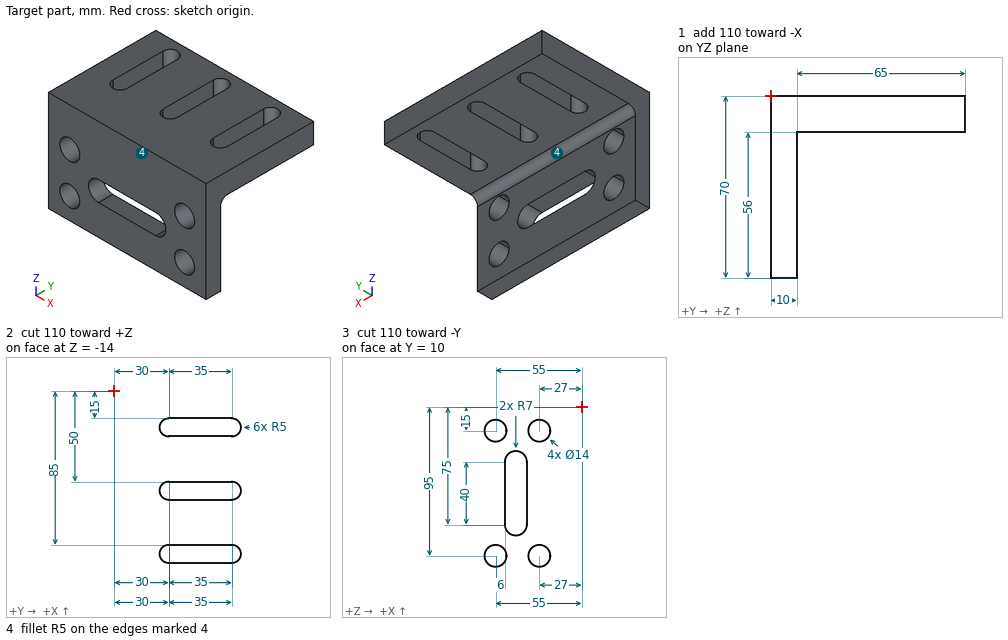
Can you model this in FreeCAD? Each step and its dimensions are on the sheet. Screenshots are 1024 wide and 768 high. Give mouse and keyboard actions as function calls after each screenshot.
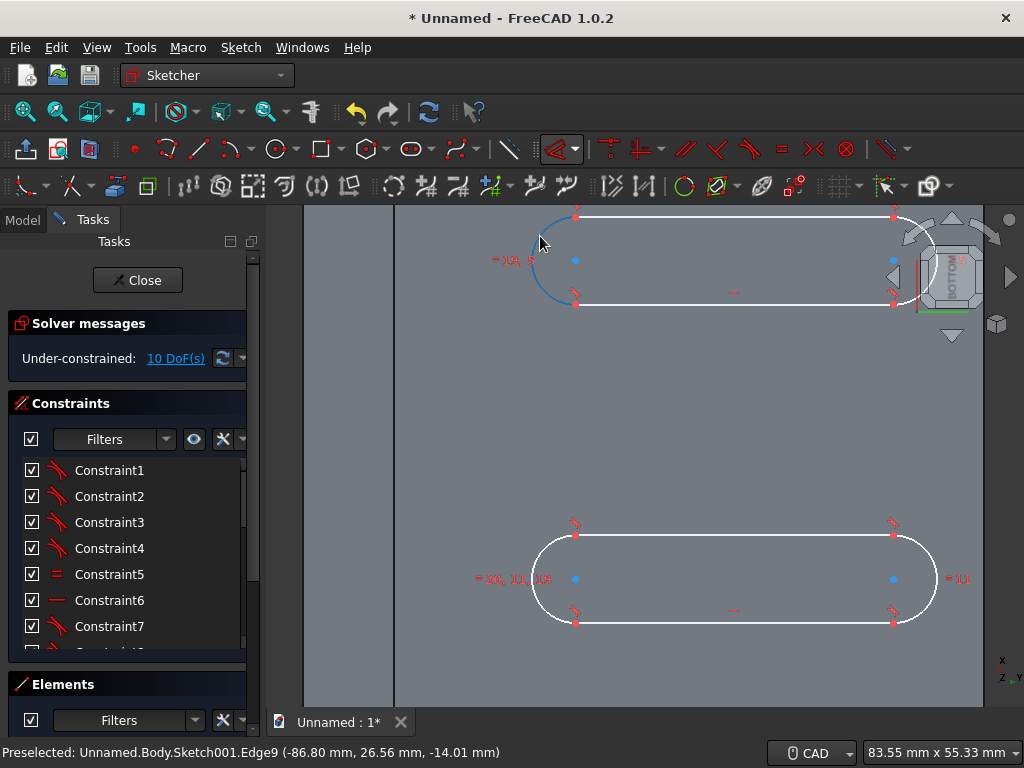
click(541, 235)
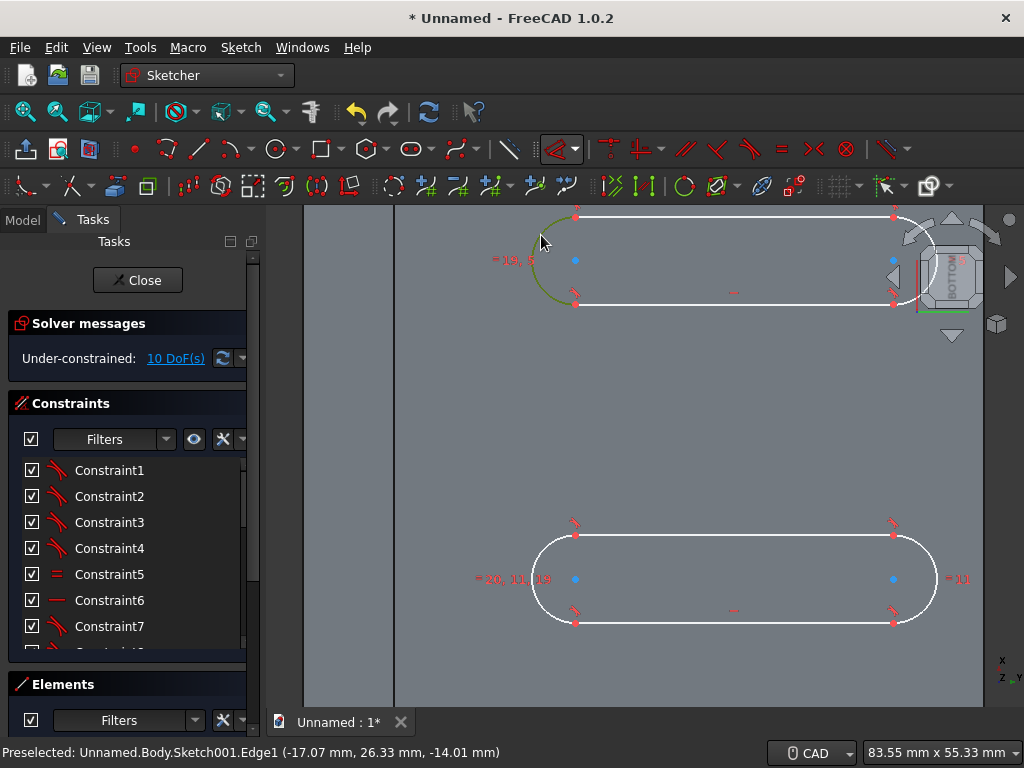
key(k)
key(r)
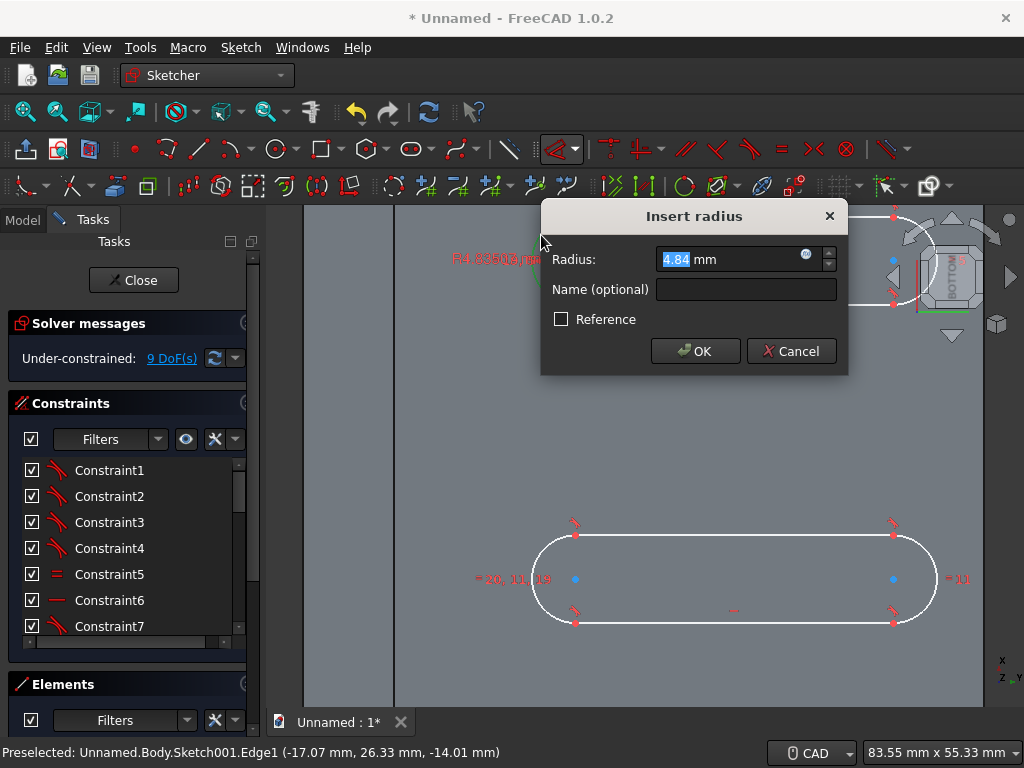
text(5)
key(Return)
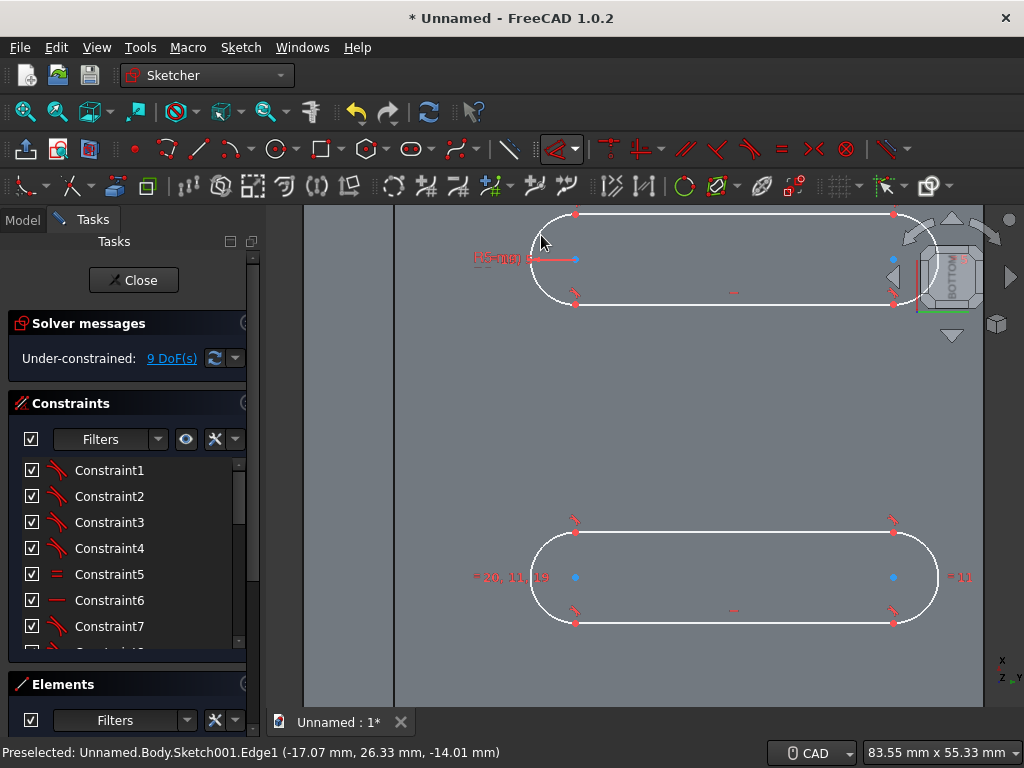
scroll(551, 425, down, 5)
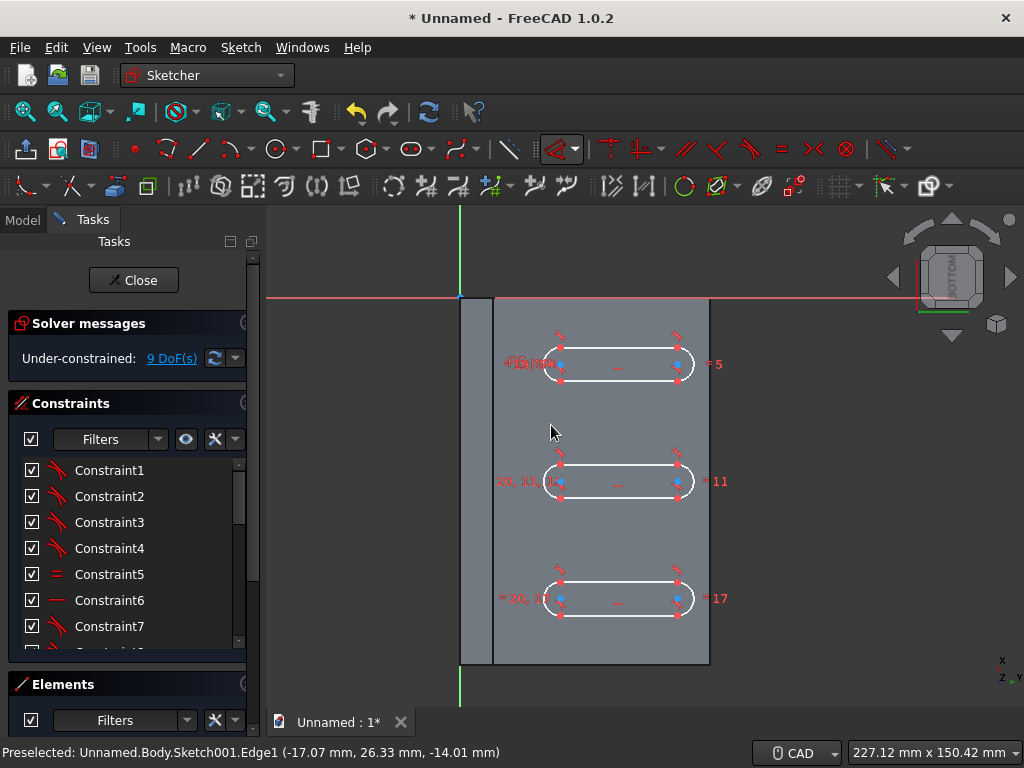
click(595, 348)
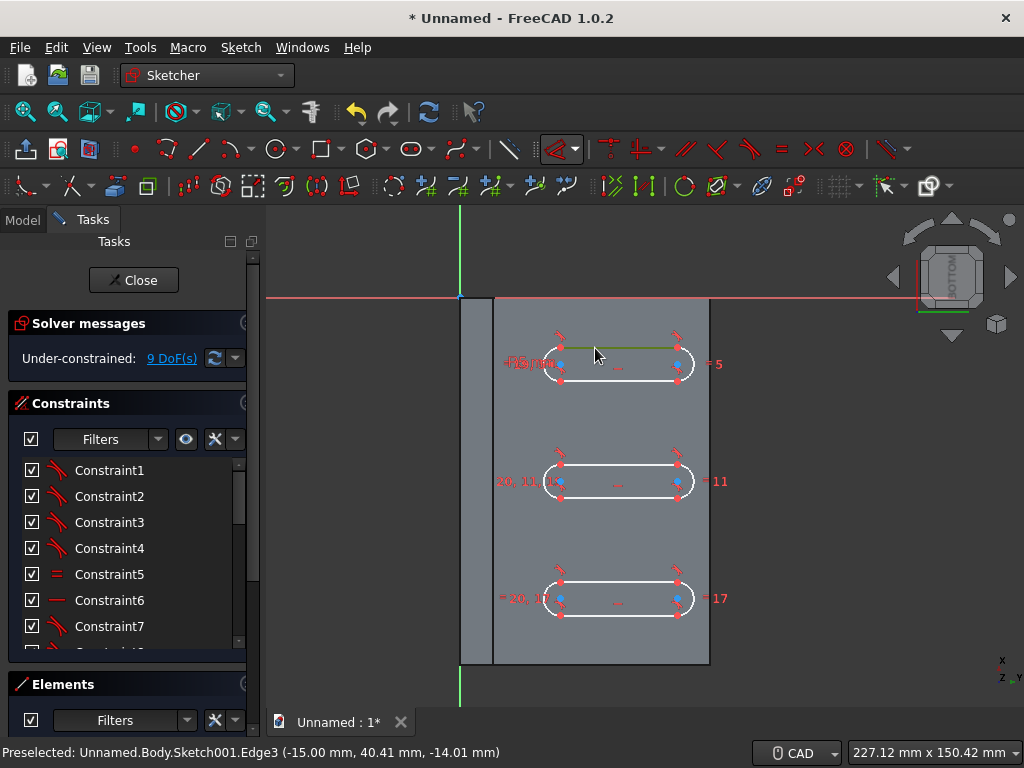
key(l)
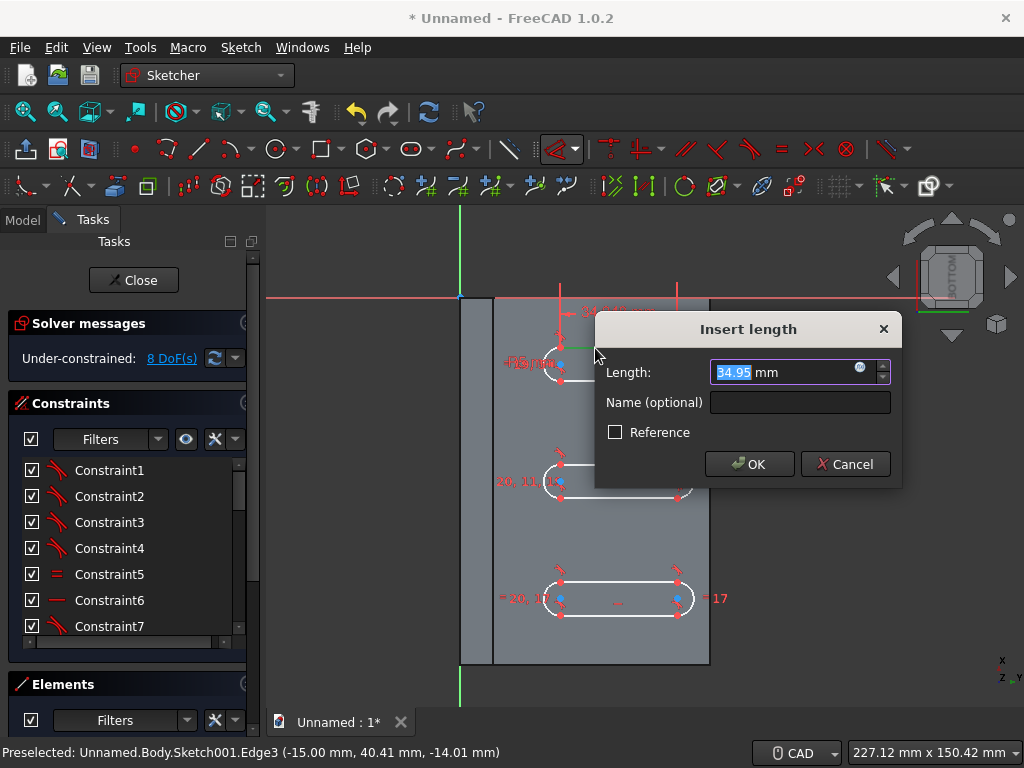
text(35)
key(Return)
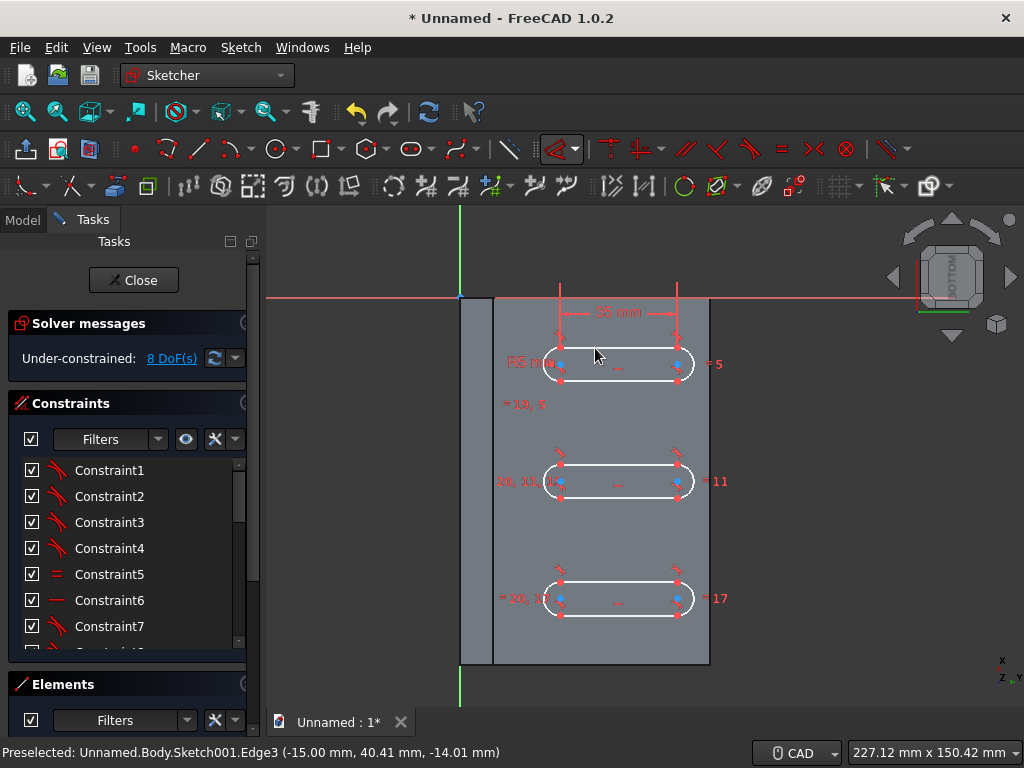
click(595, 465)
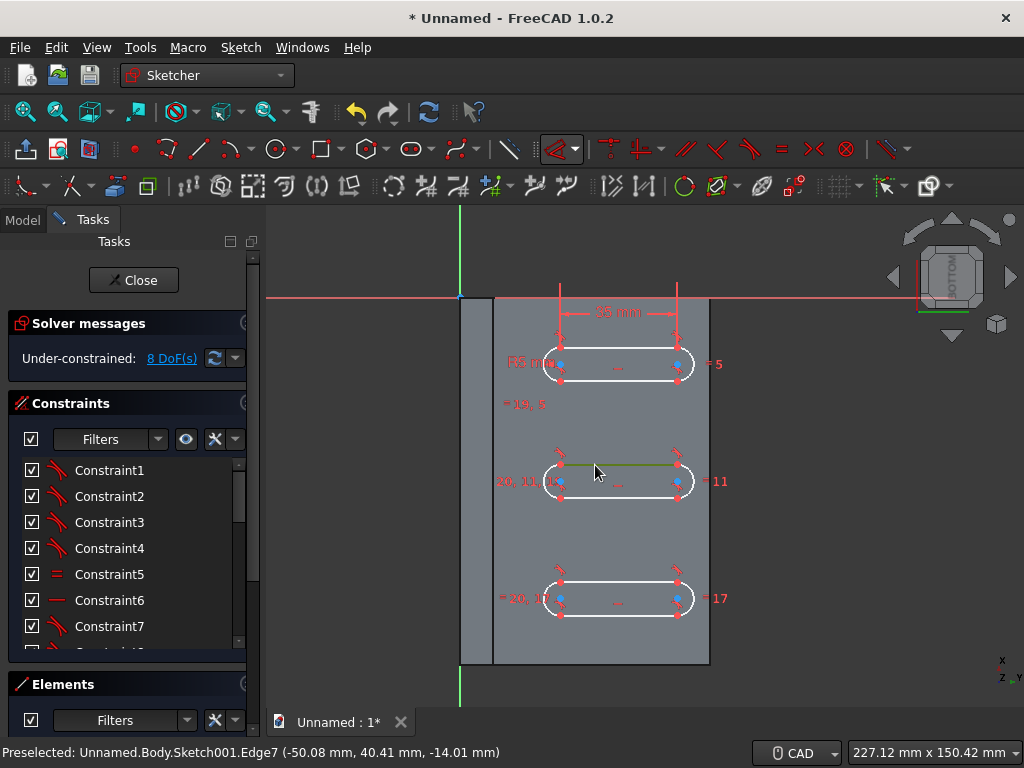
key(l)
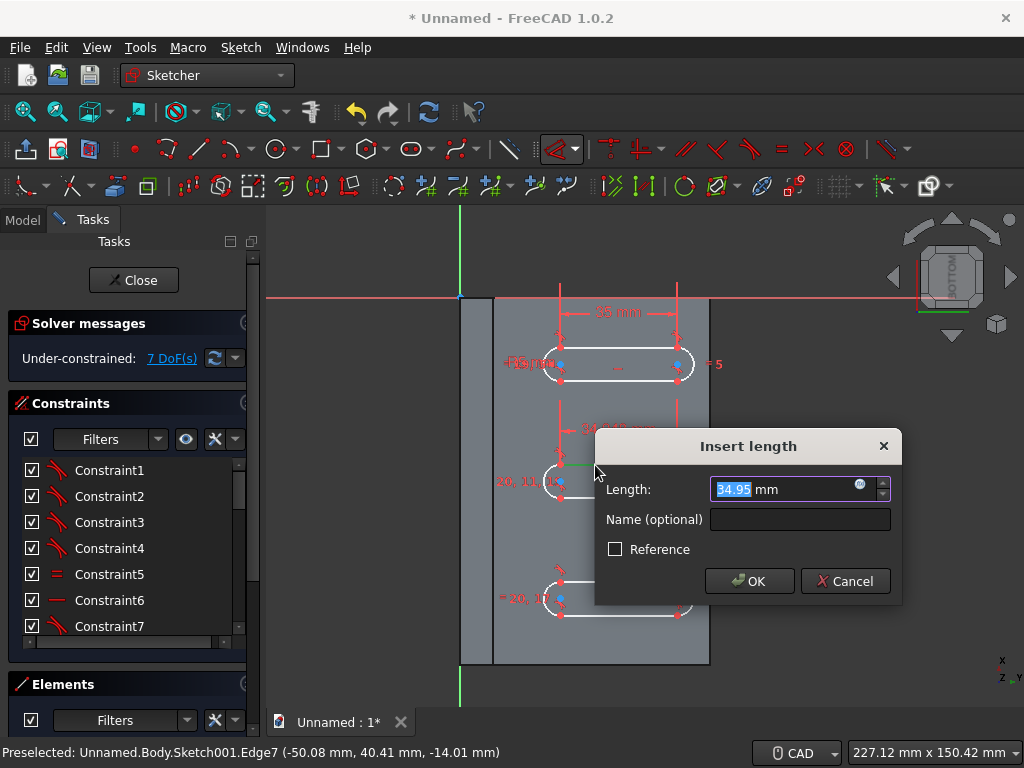
text(35)
key(Return)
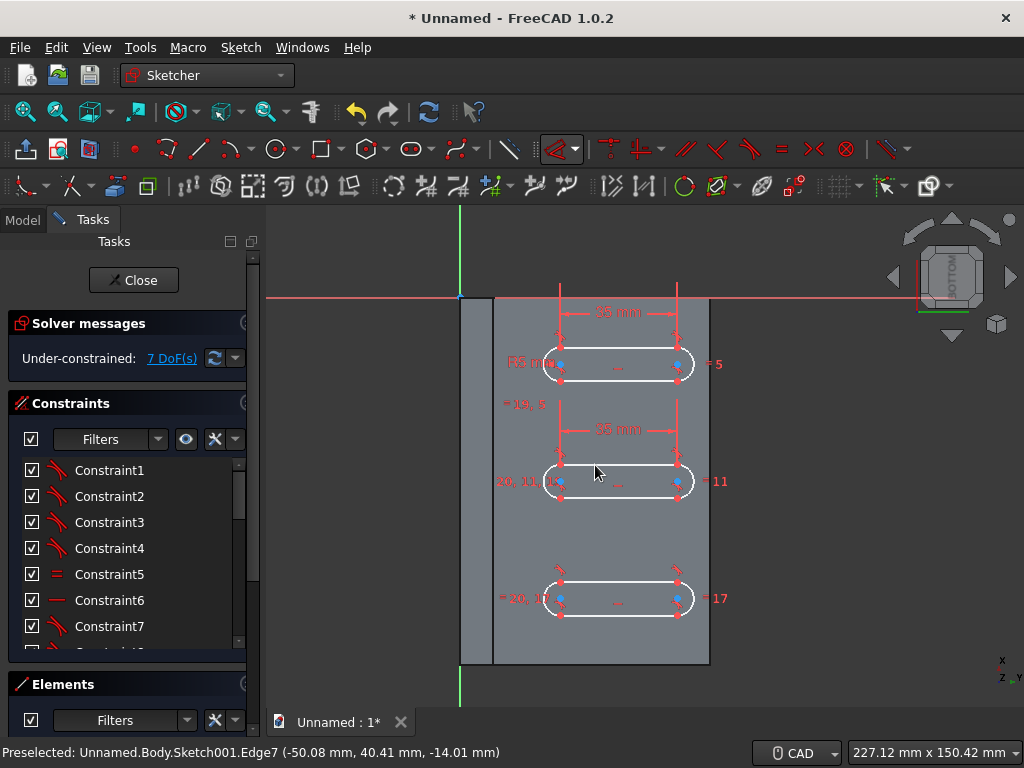
click(595, 582)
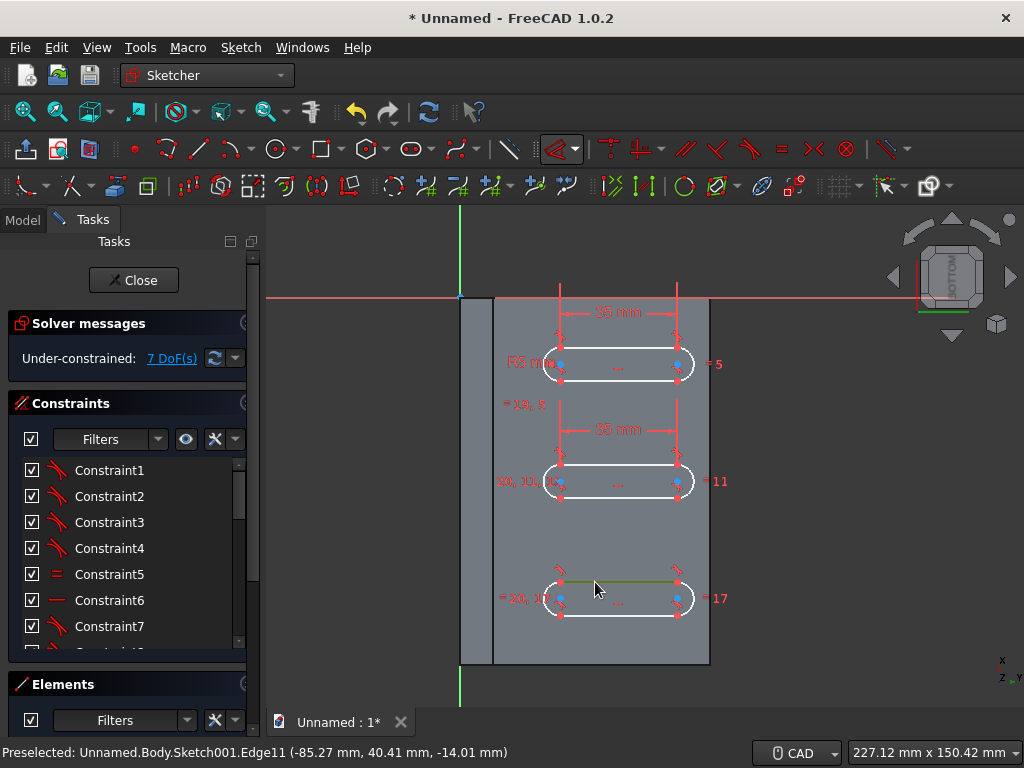
key(l)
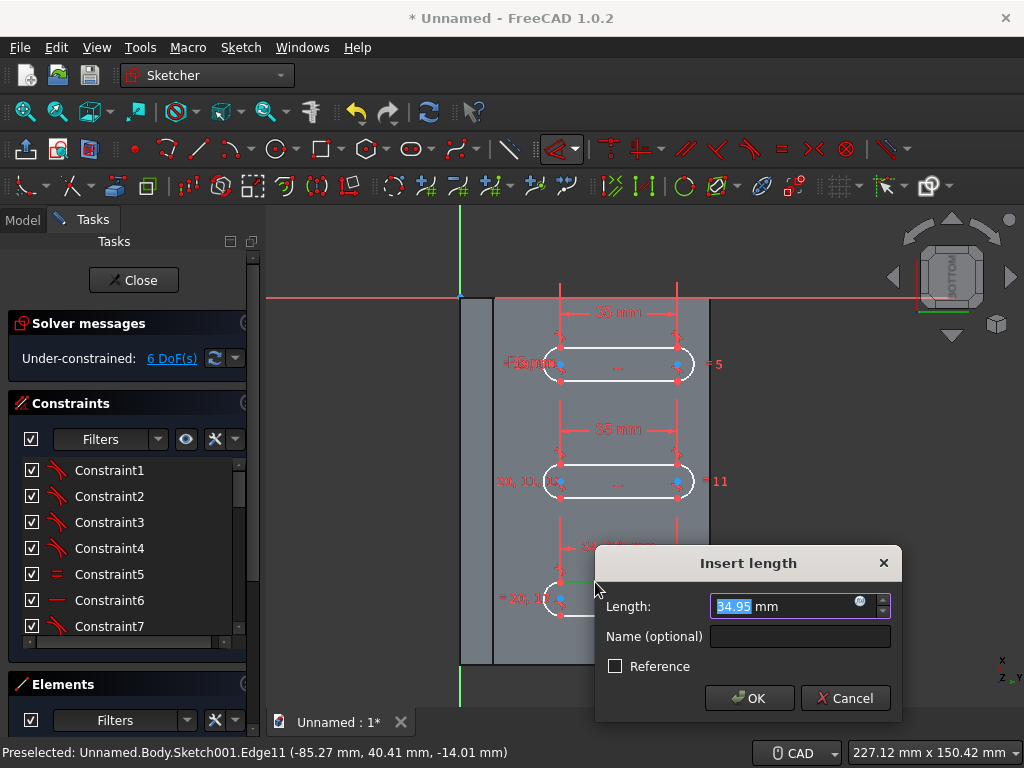
text(35)
key(Return)